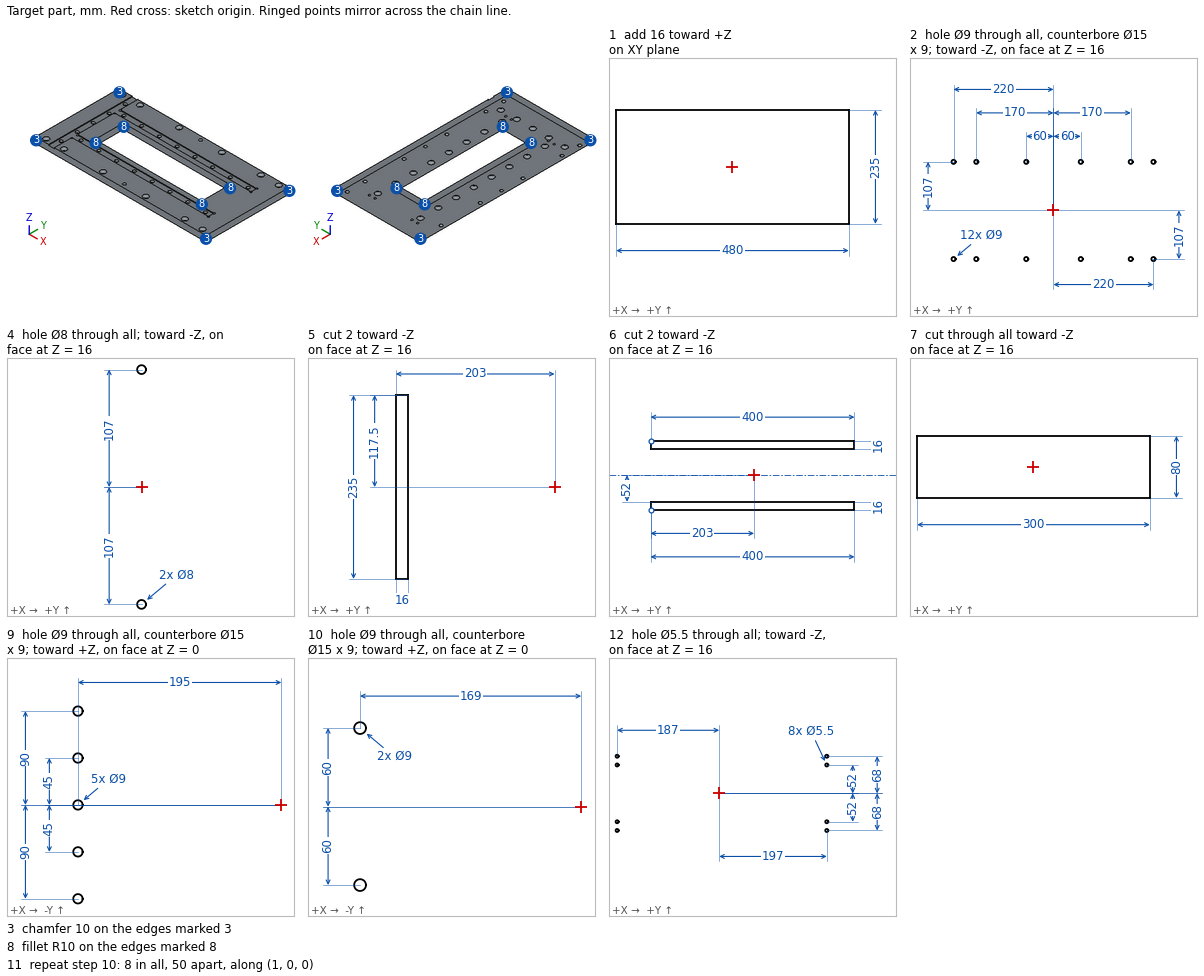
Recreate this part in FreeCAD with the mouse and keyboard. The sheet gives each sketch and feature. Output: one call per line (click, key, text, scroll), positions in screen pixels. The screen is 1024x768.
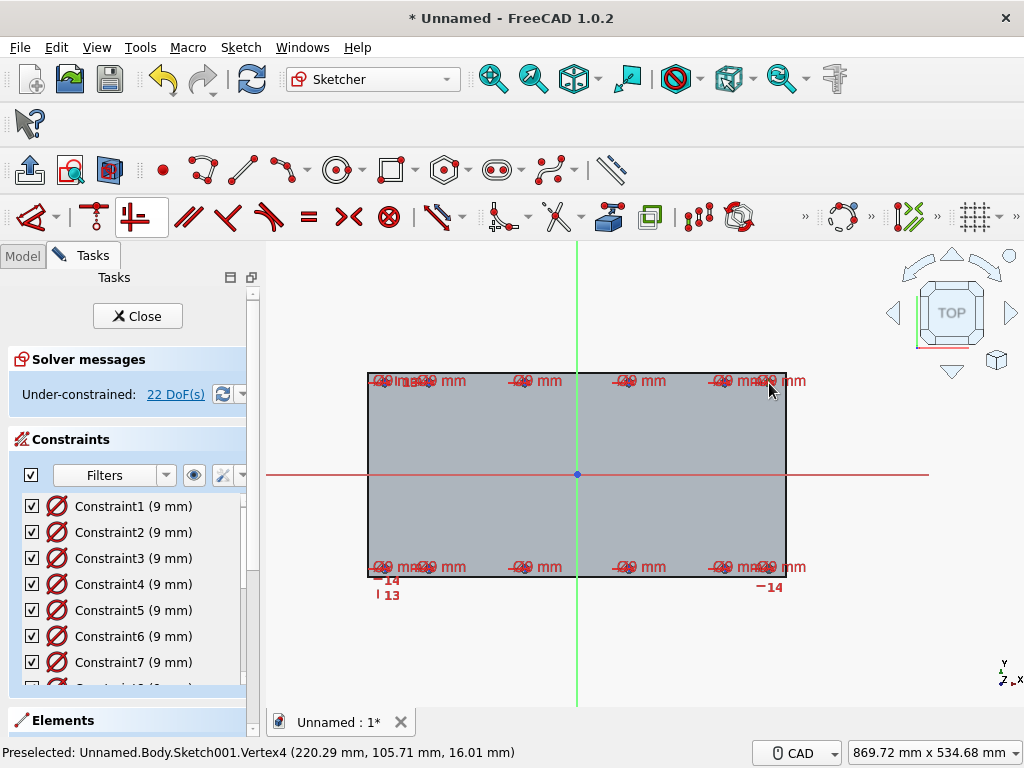
click(162, 218)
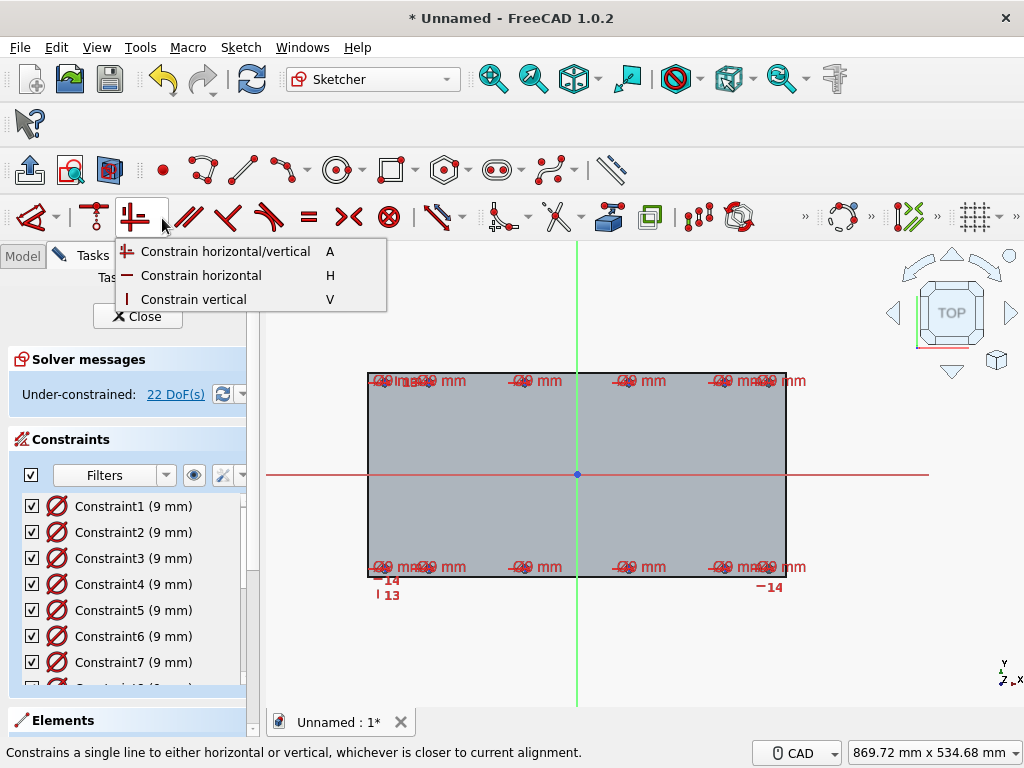
click(251, 299)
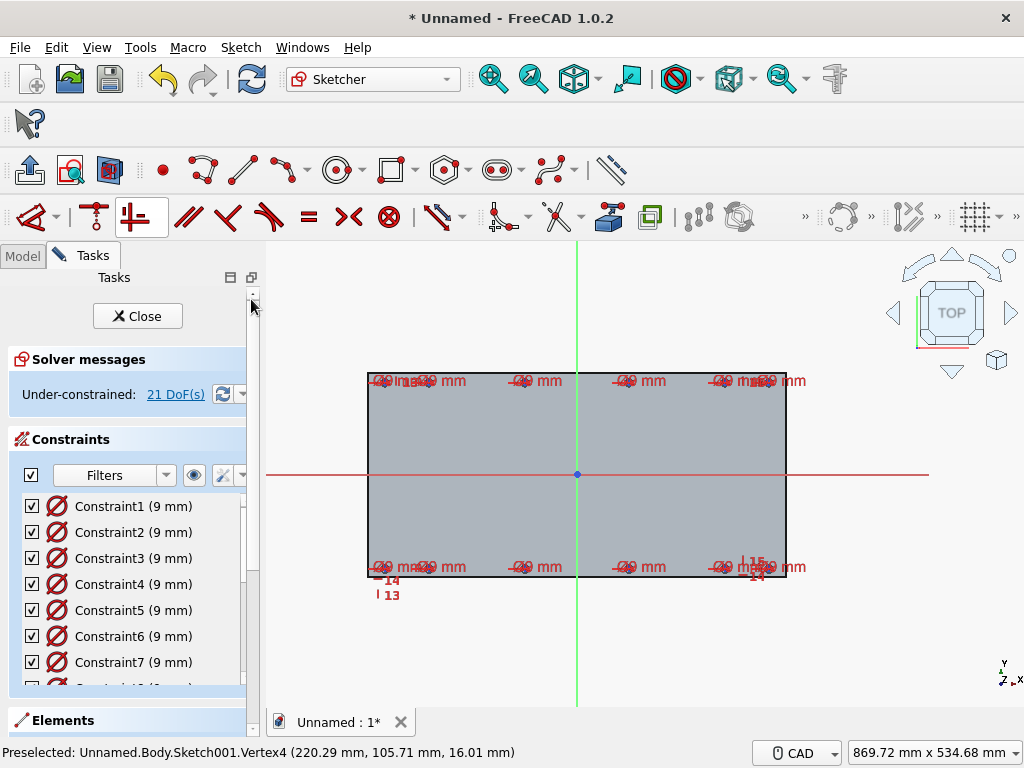
click(385, 383)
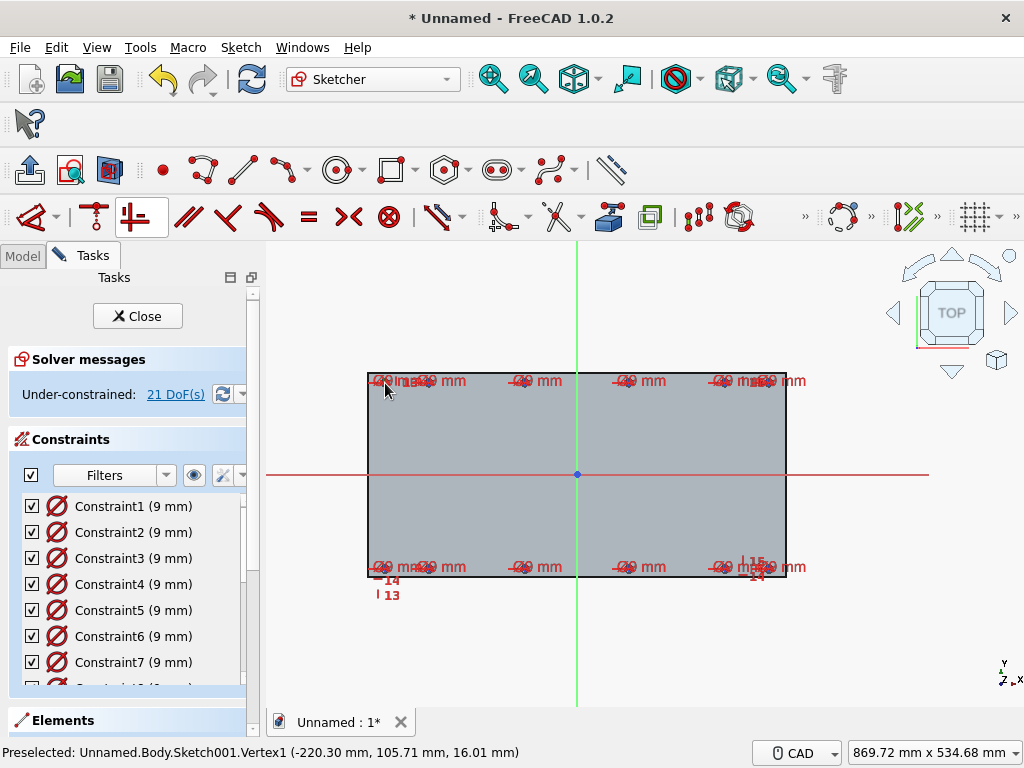
click(769, 383)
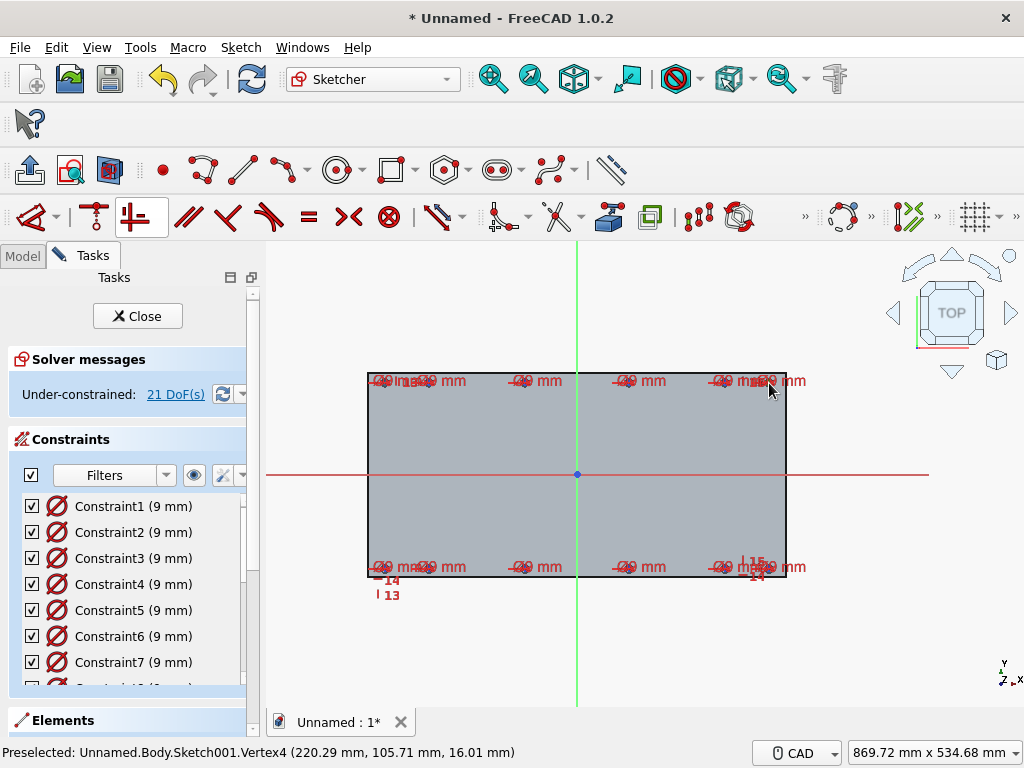
click(162, 218)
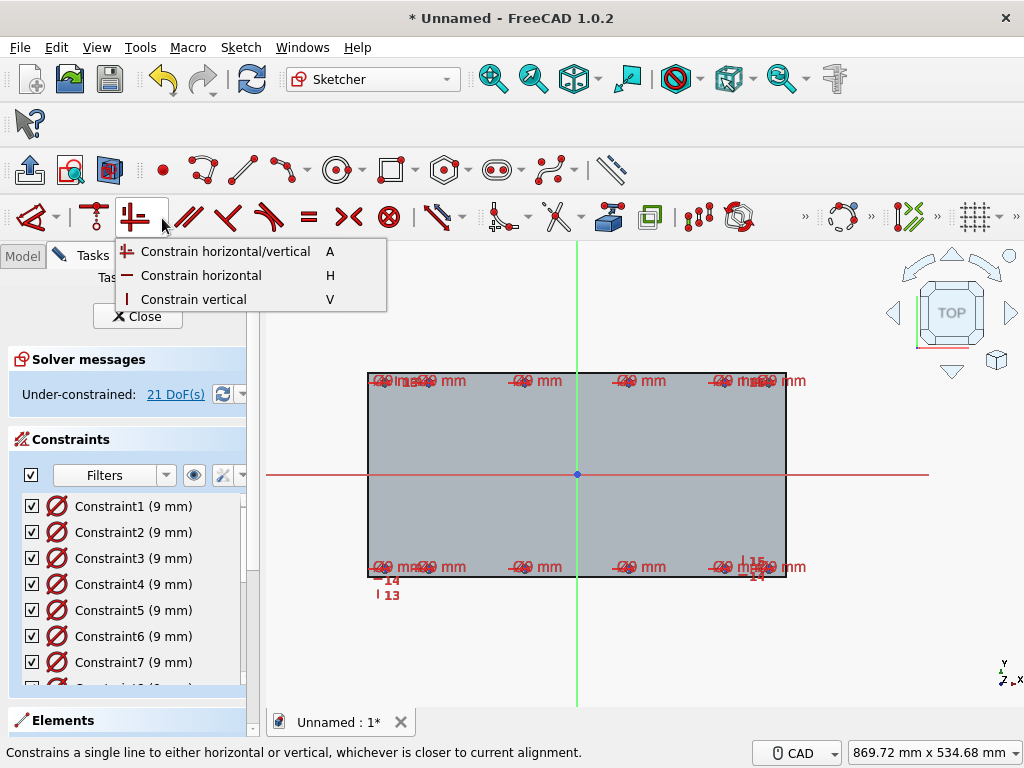
click(251, 275)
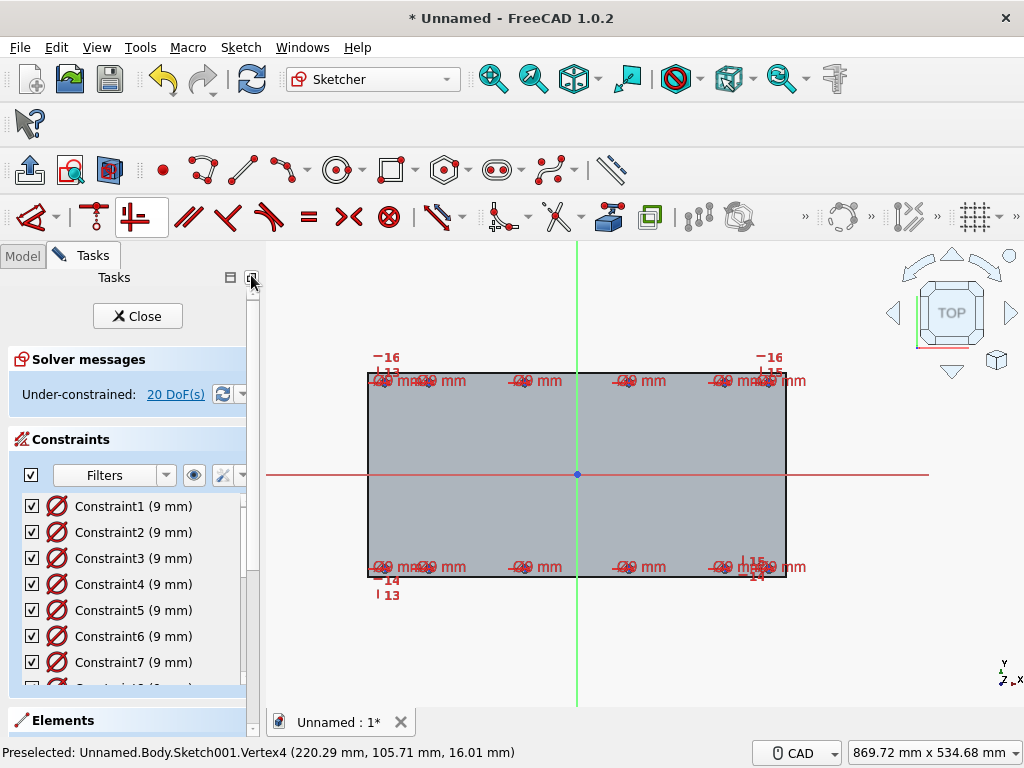
click(385, 383)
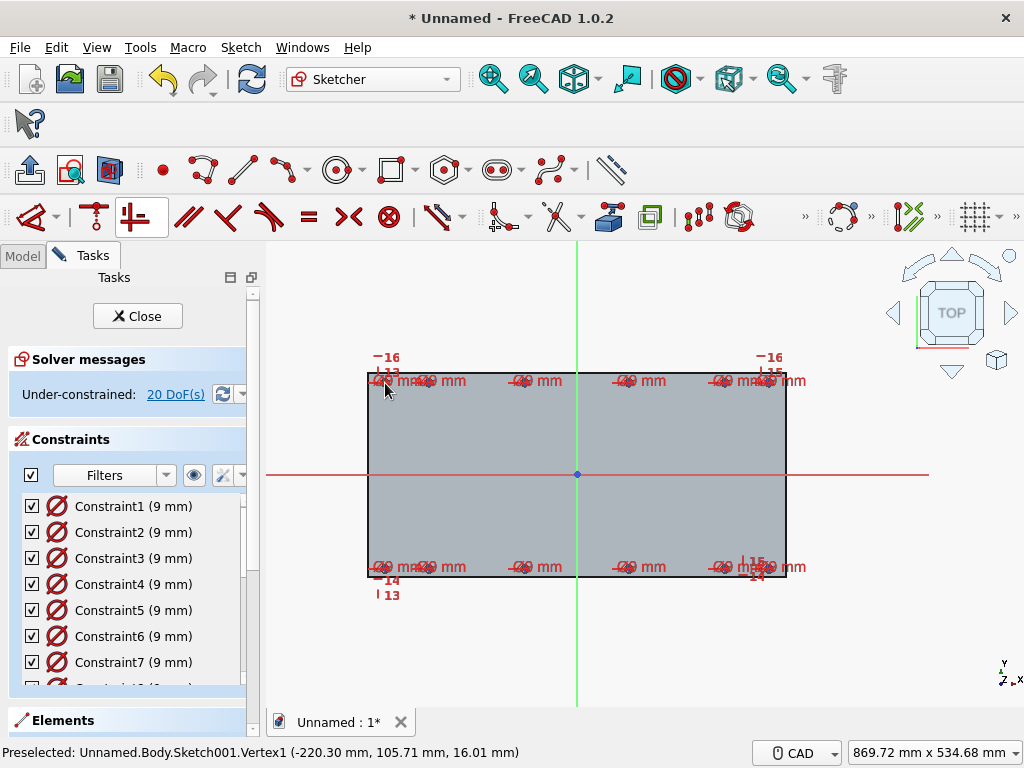
click(429, 383)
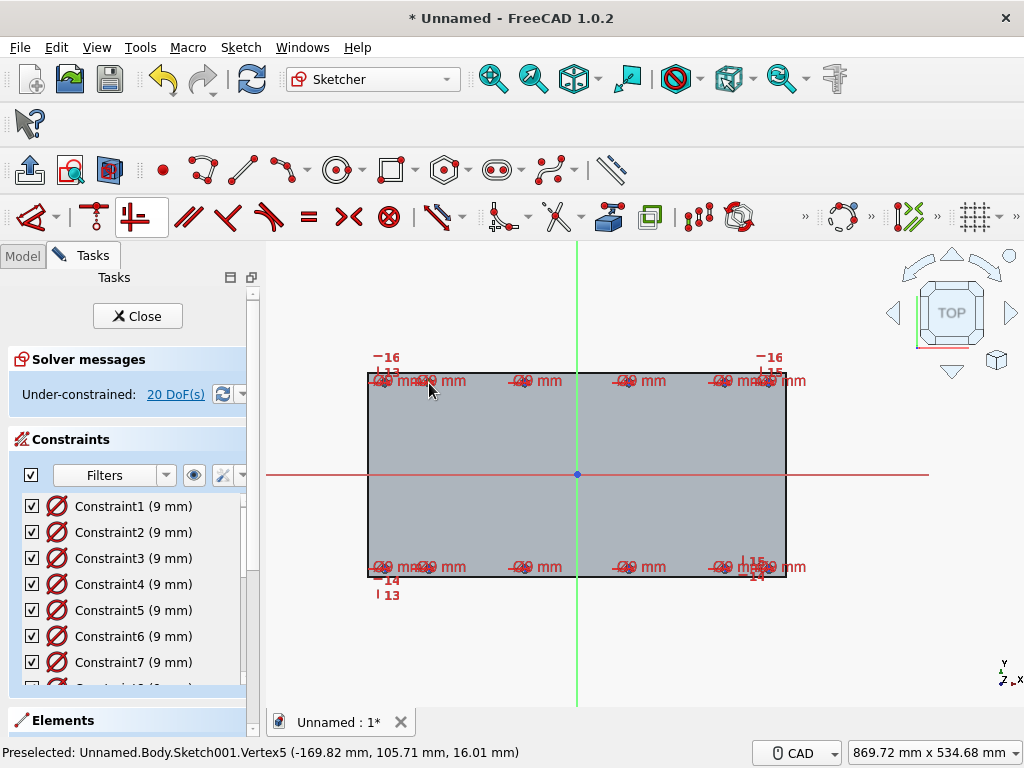
key(h)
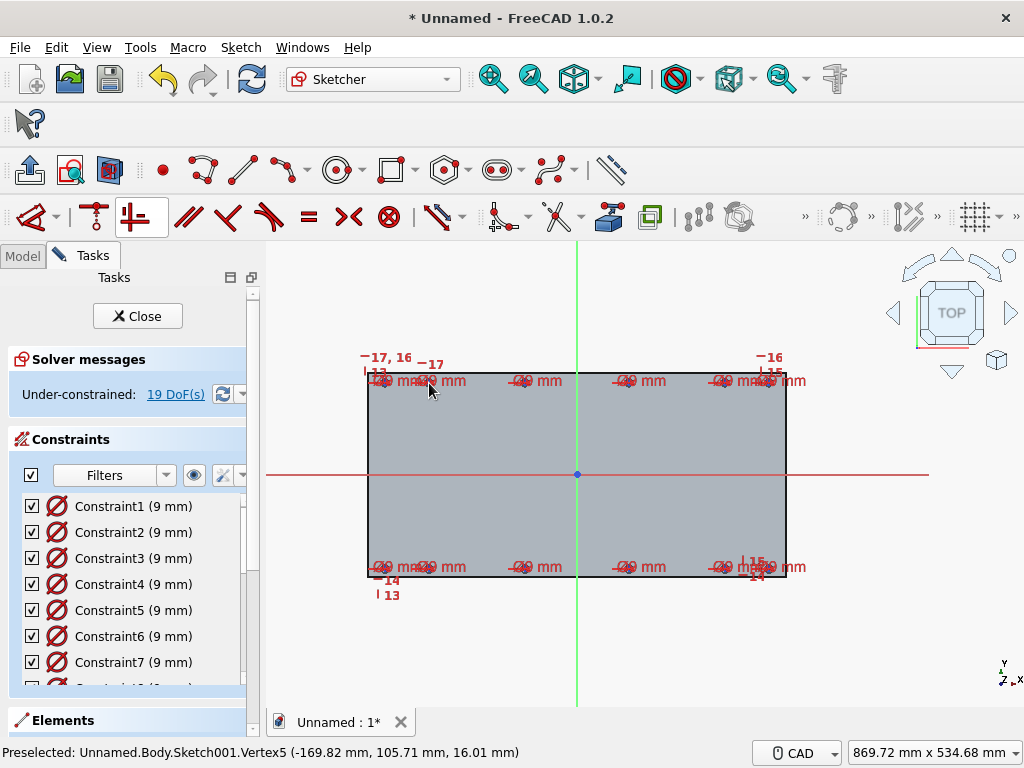
click(429, 383)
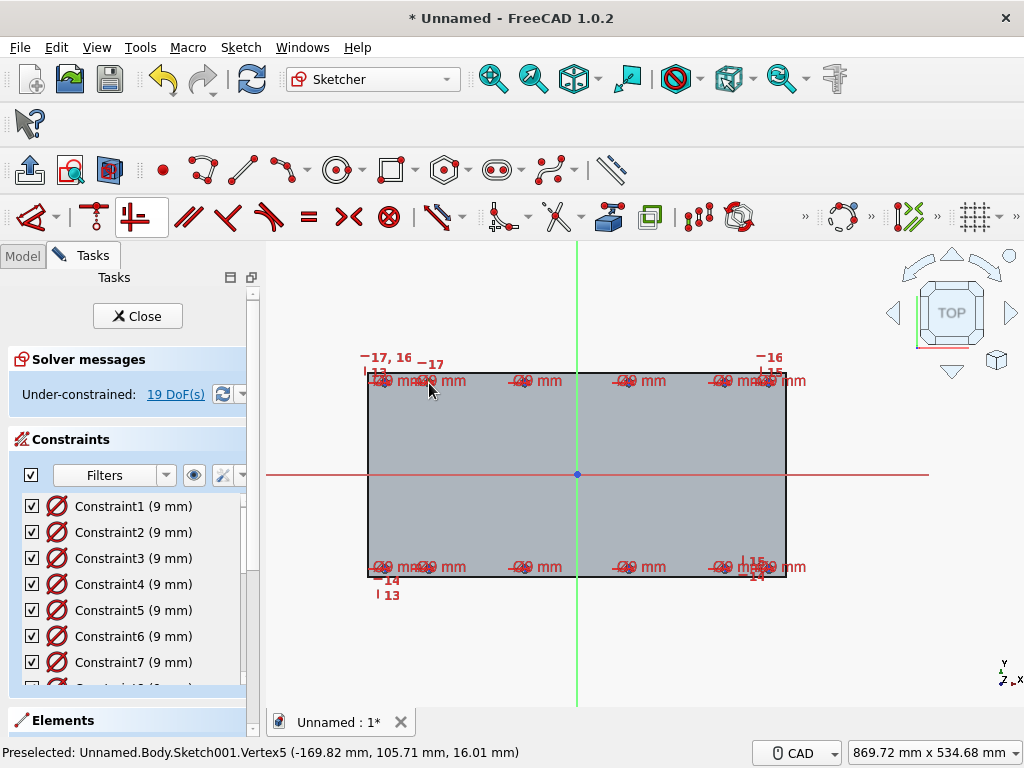
click(429, 569)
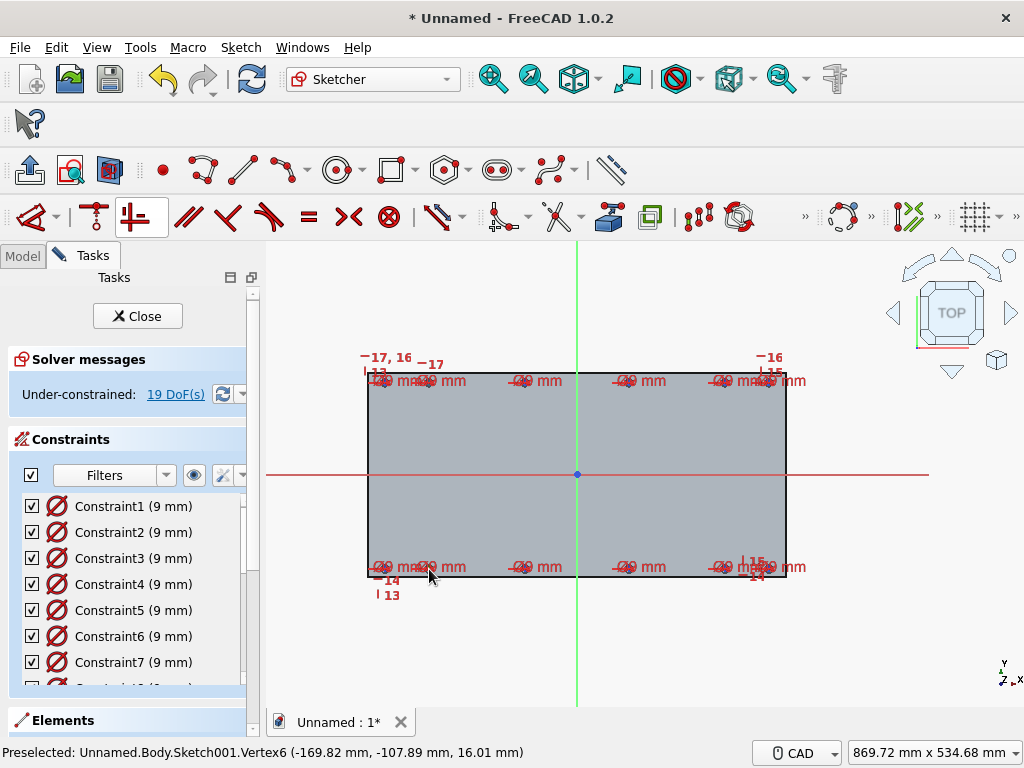
click(162, 218)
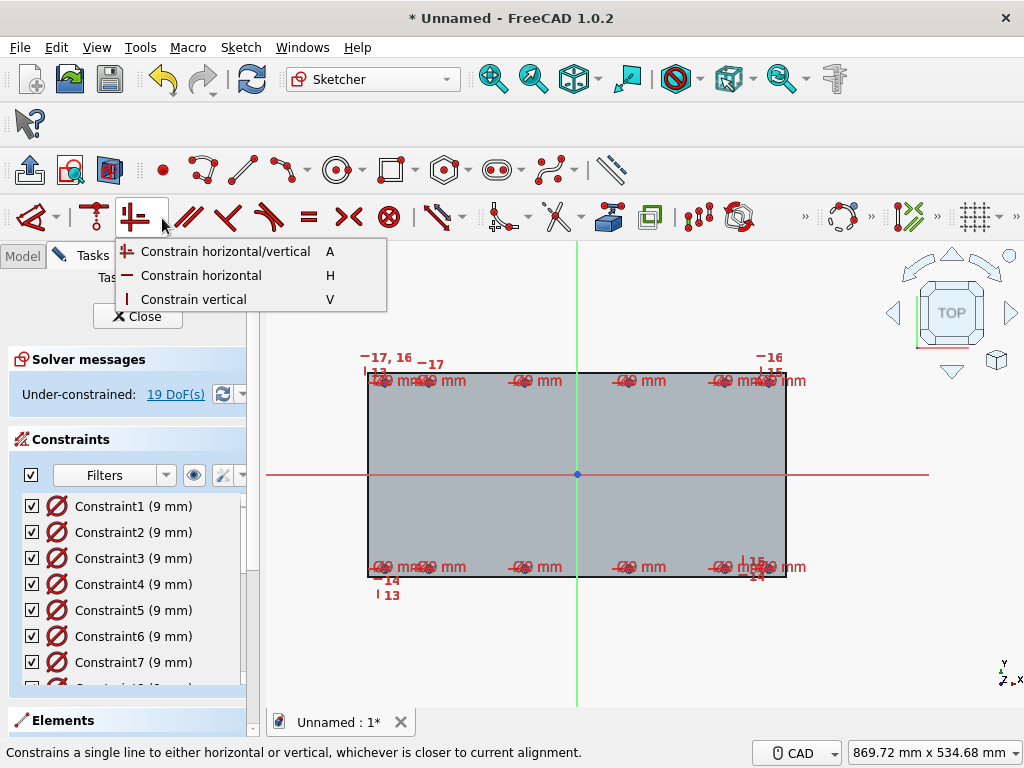
click(251, 299)